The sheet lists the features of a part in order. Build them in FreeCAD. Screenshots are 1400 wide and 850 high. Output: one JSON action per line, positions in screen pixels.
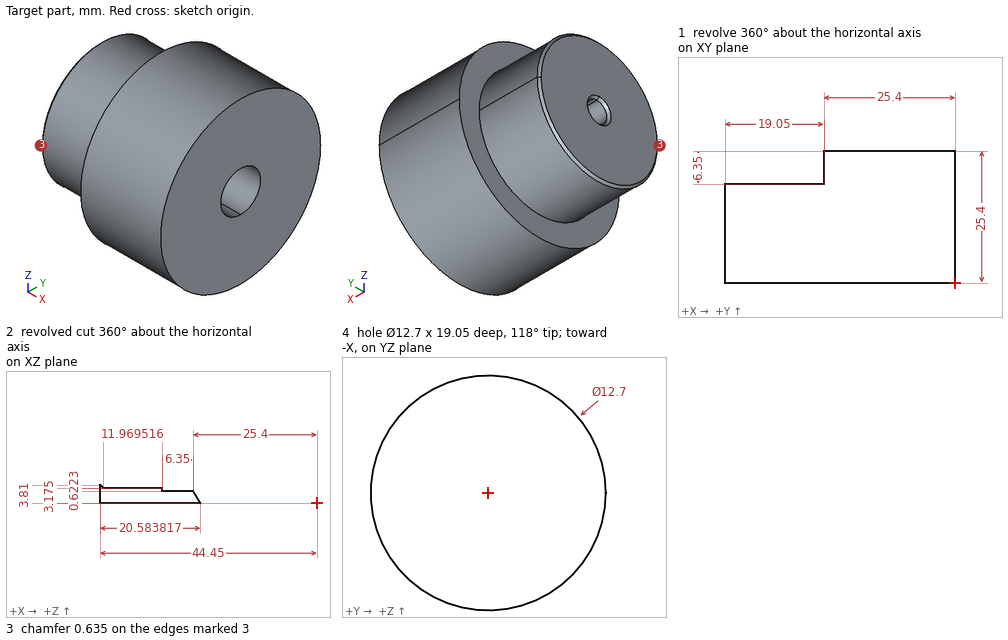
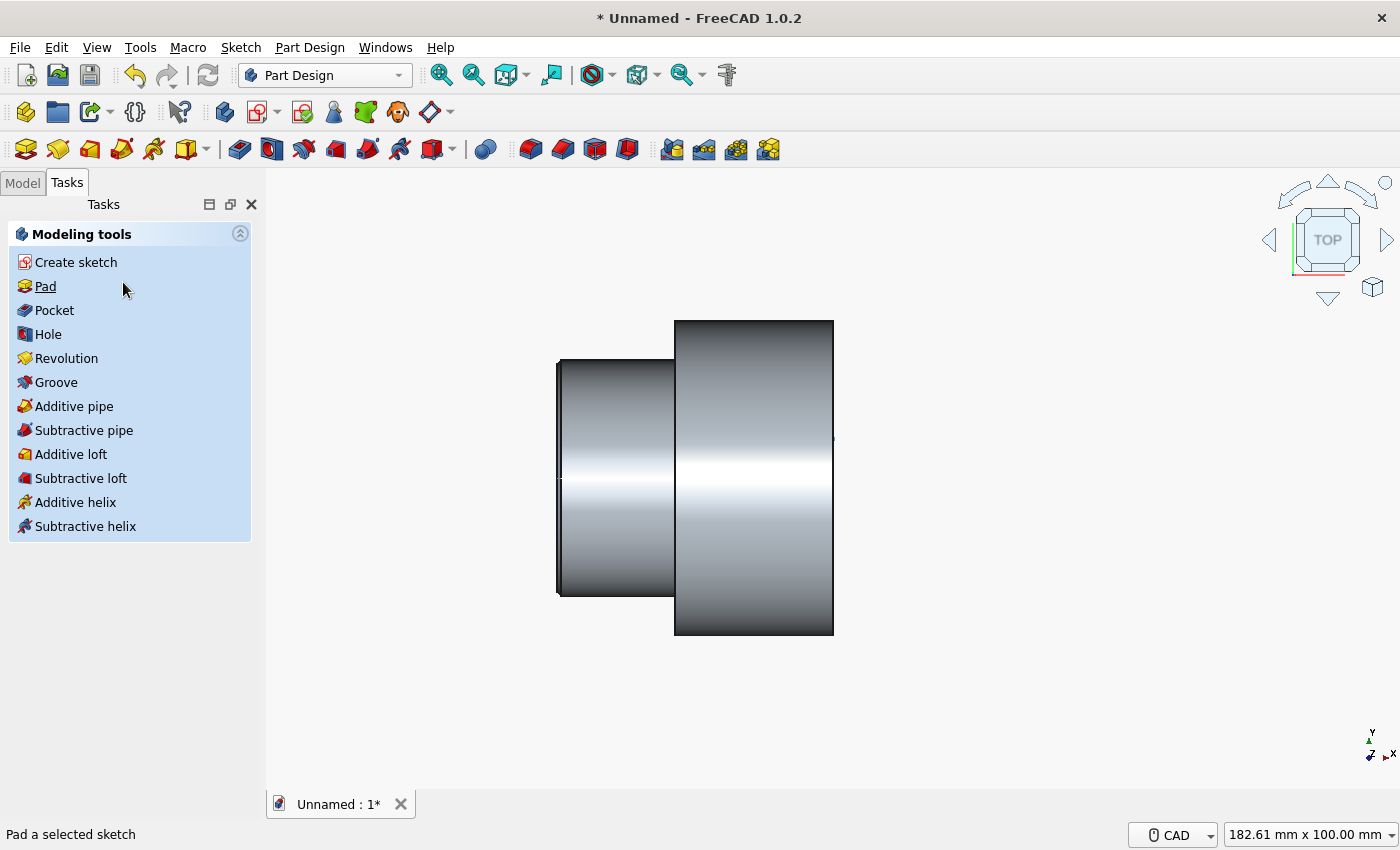
{"action": "left_click", "coordinate": [272, 150]}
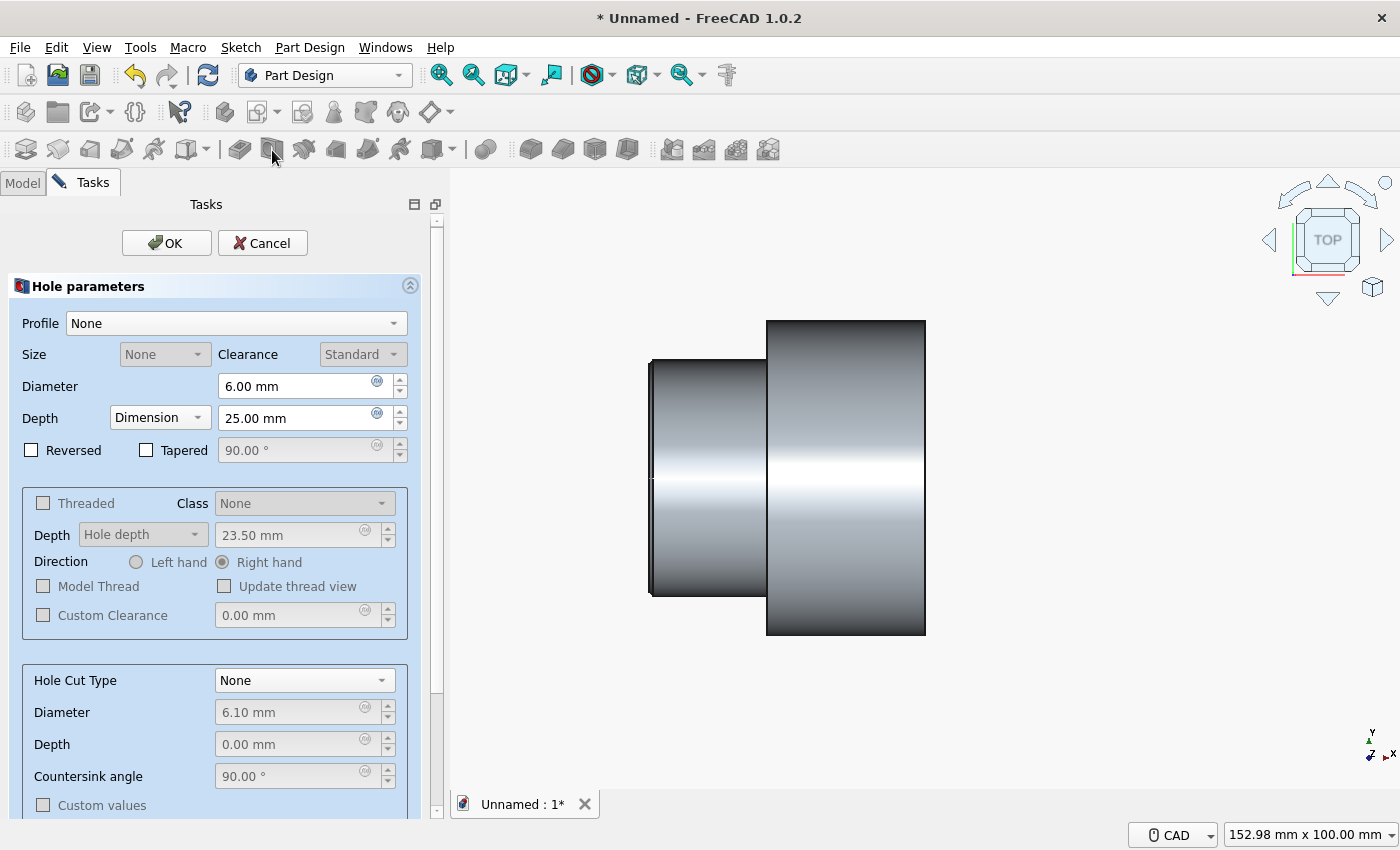
{"action": "triple_click", "coordinate": [305, 386]}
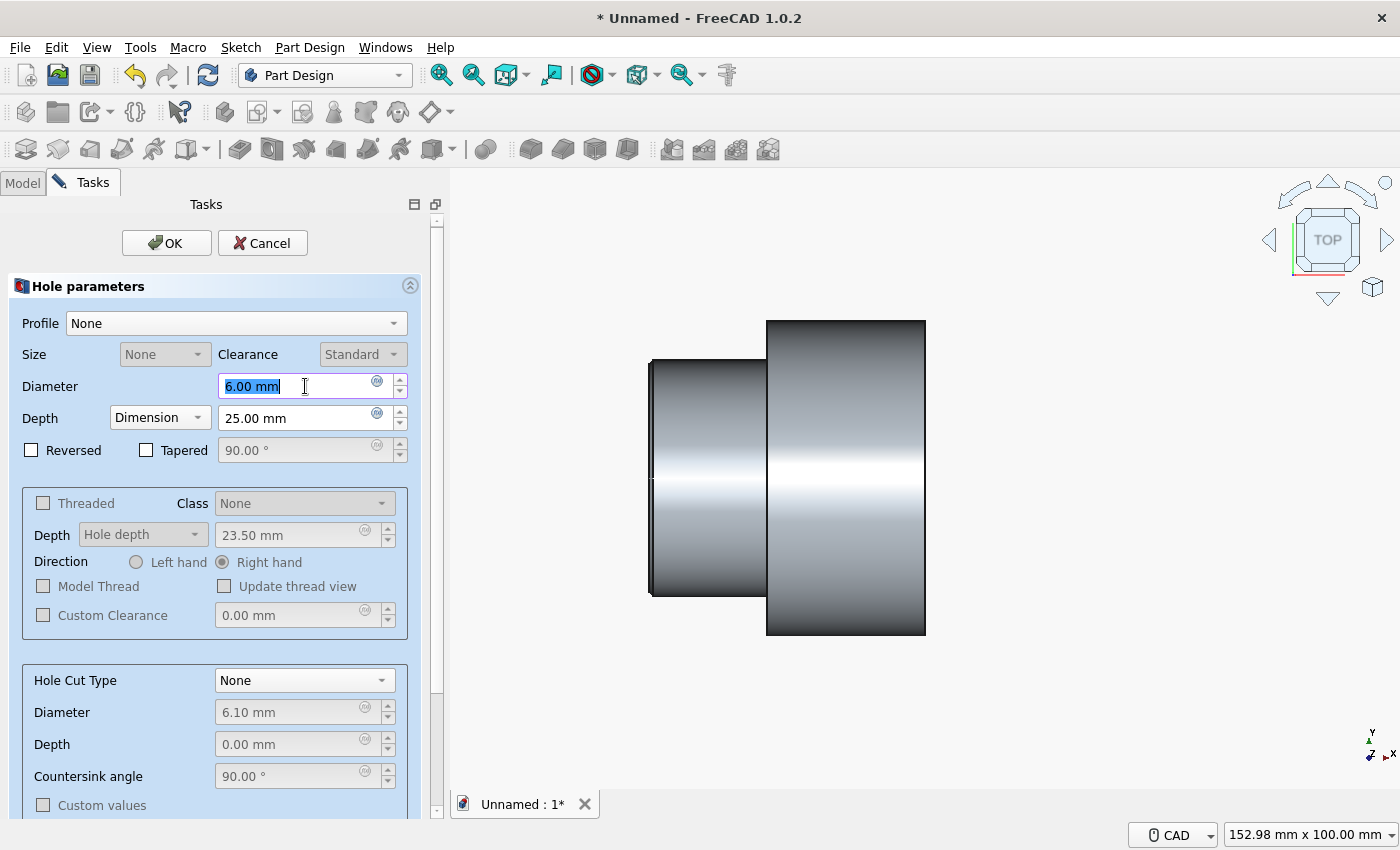
{"action": "type", "text": "12.7"}
{"action": "key", "text": "Tab"}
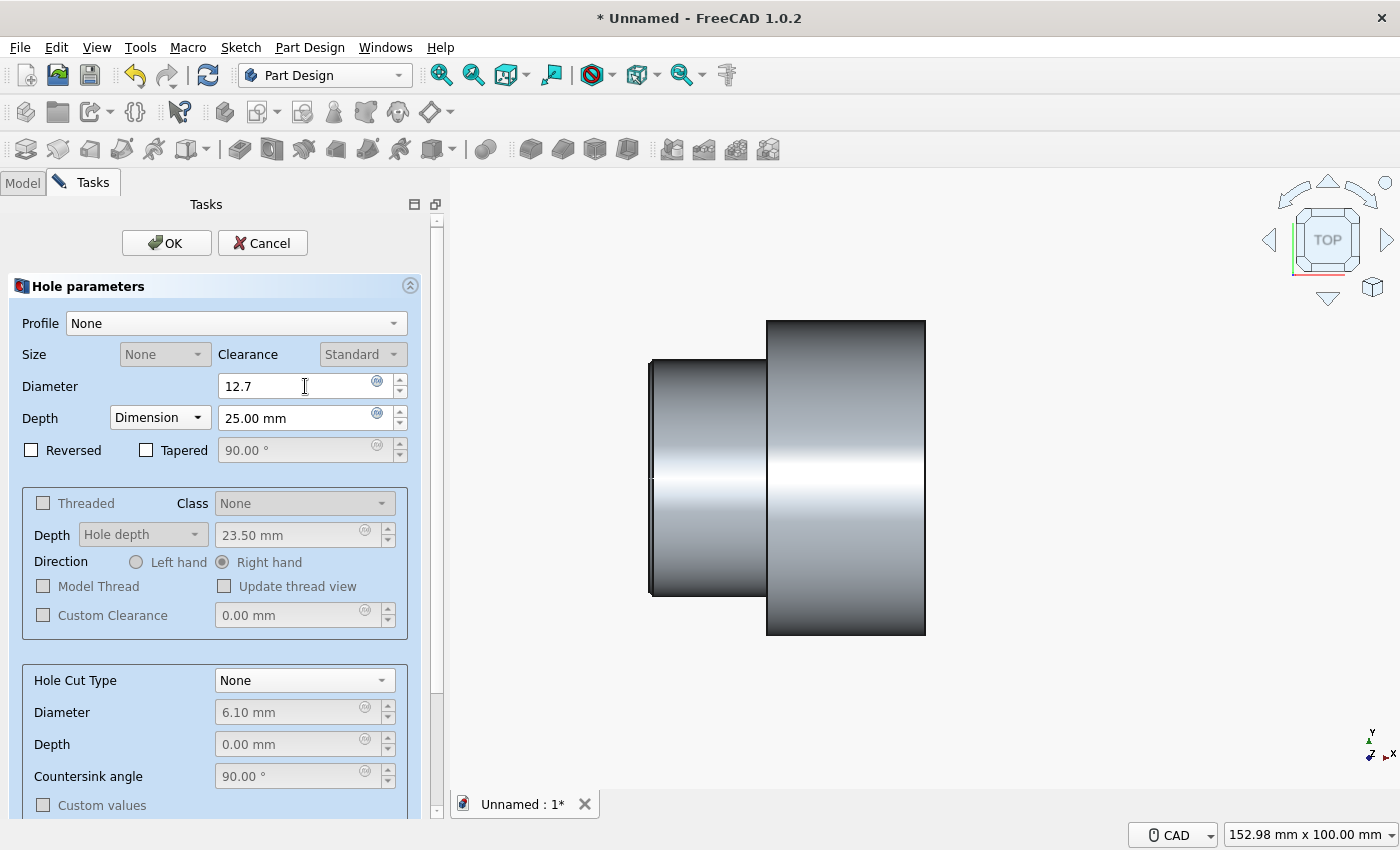
{"action": "triple_click", "coordinate": [305, 418]}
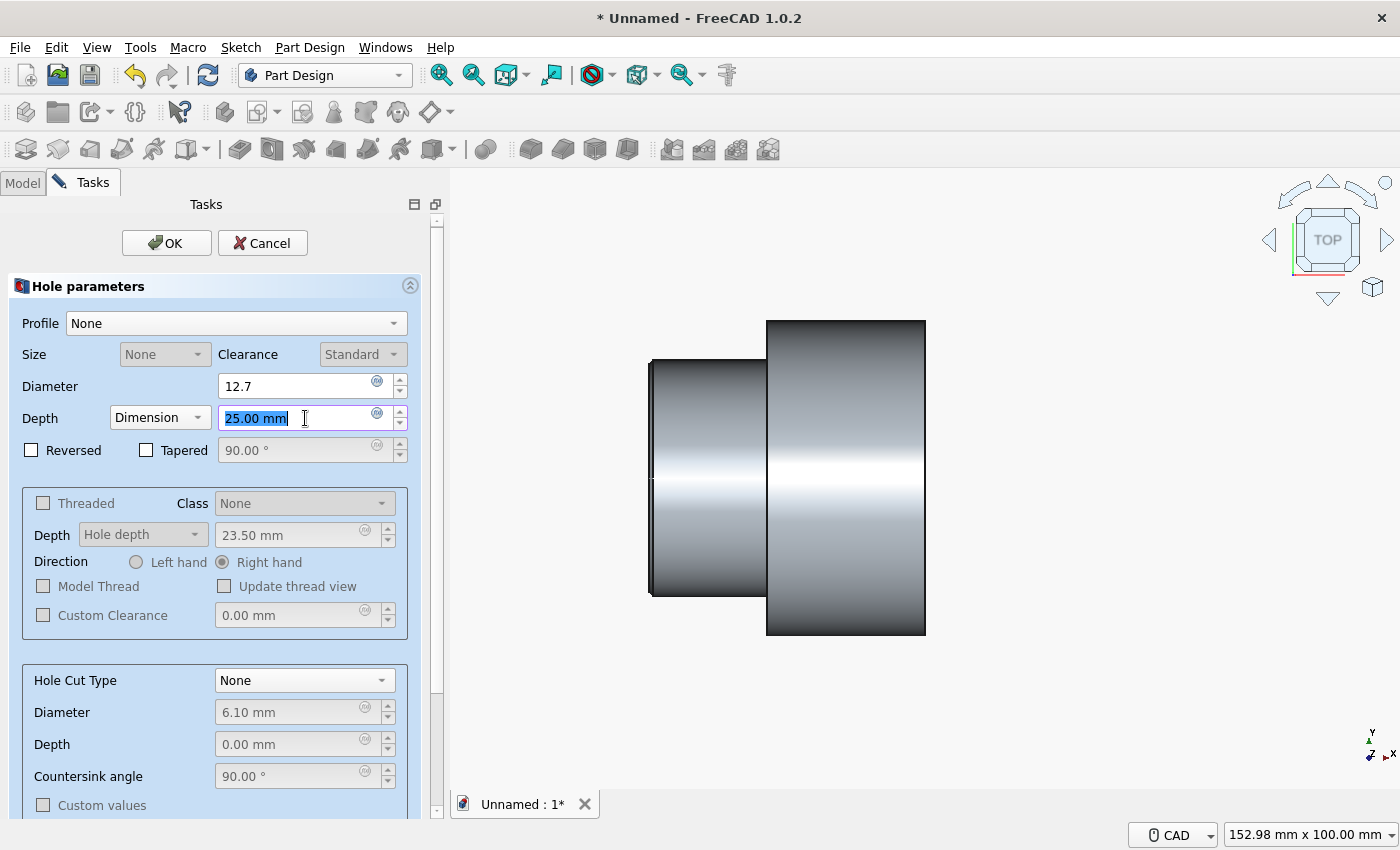
{"action": "type", "text": "19.05"}
{"action": "key", "text": "Tab"}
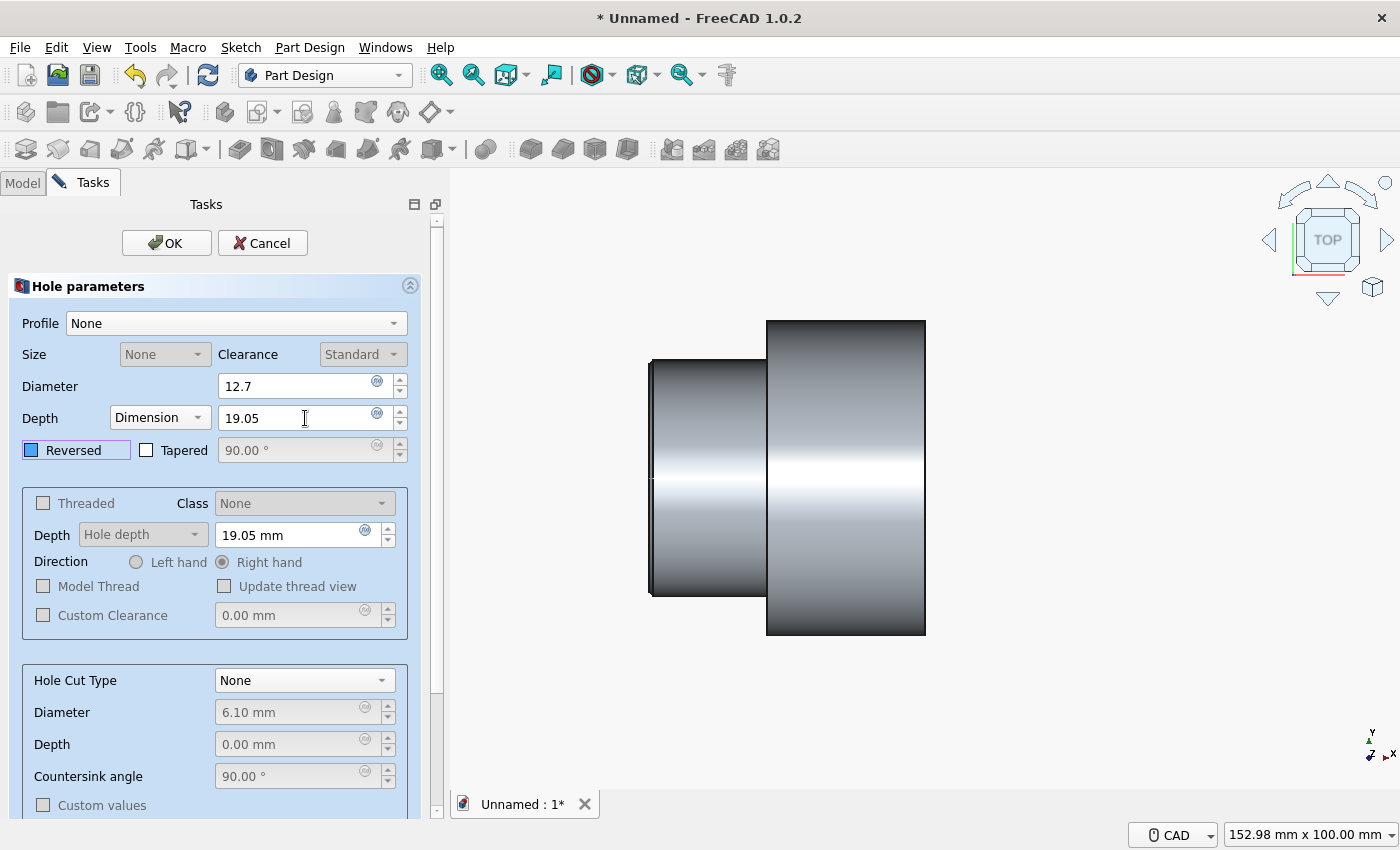
{"action": "left_click", "coordinate": [167, 243]}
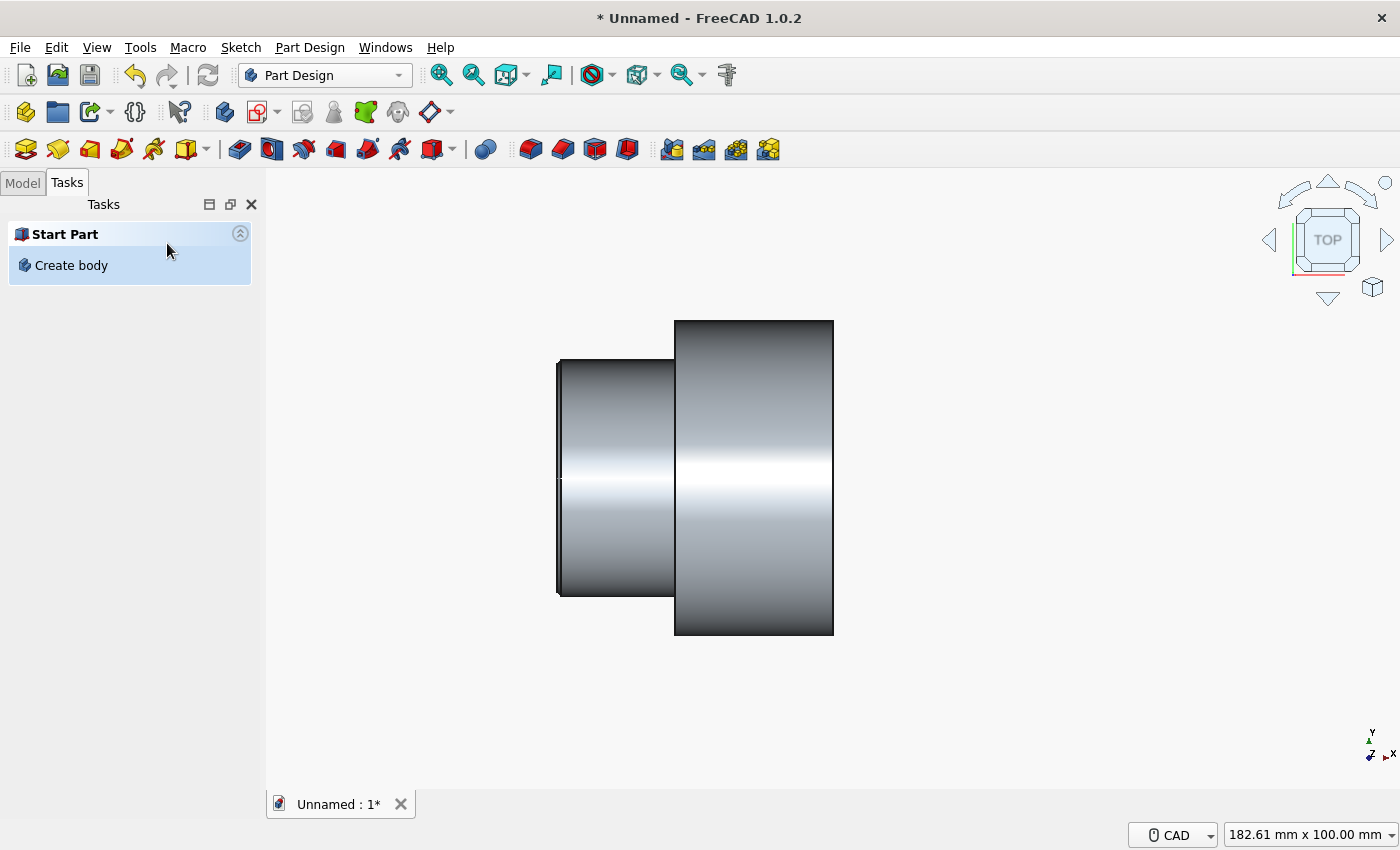
{"action": "key", "text": "0"}